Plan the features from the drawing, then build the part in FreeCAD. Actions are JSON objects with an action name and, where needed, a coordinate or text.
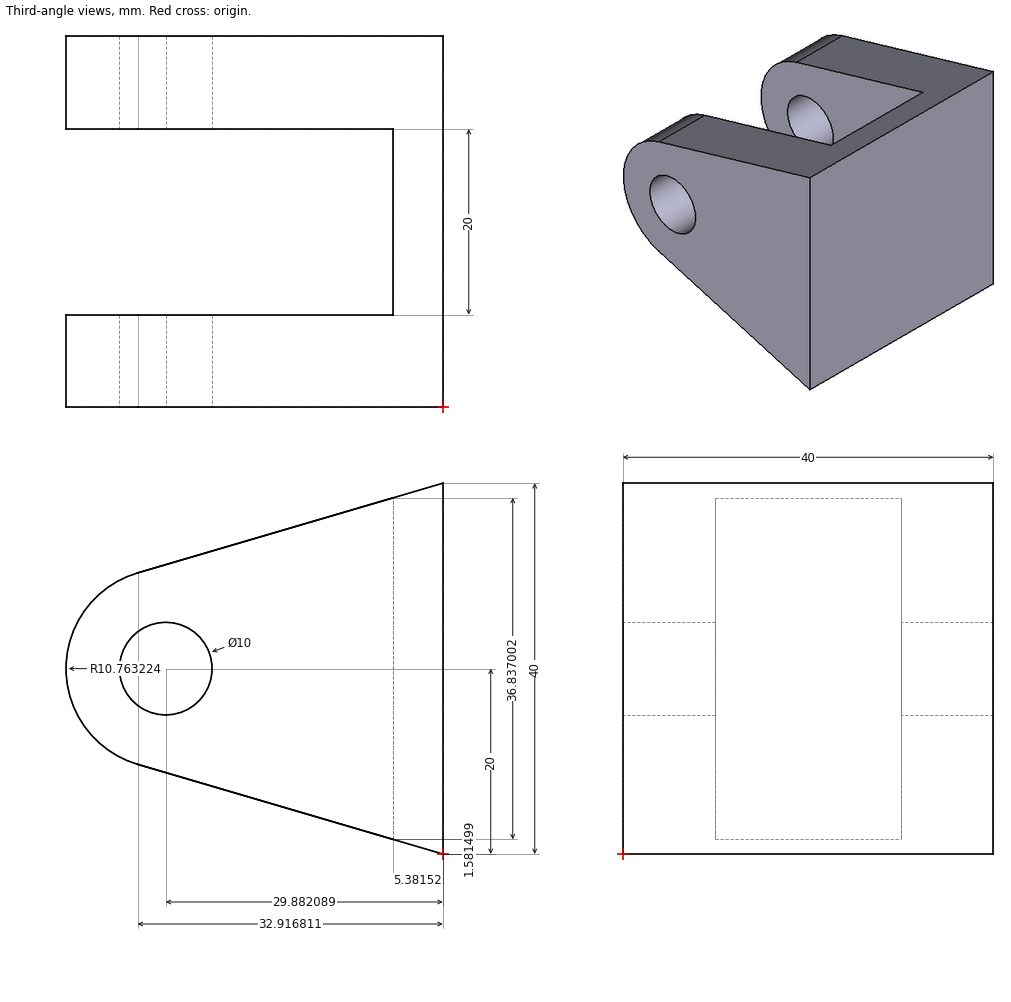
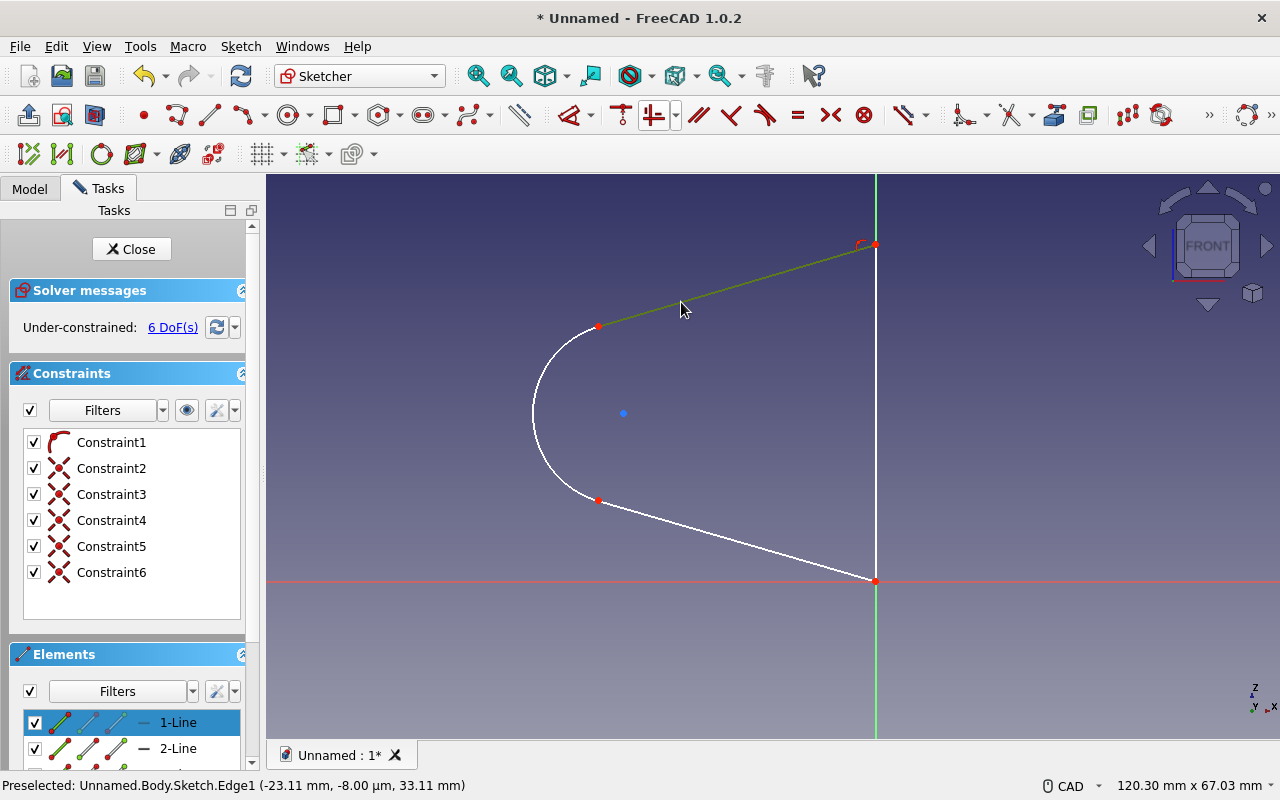
{"action": "left_click", "coordinate": [545, 369]}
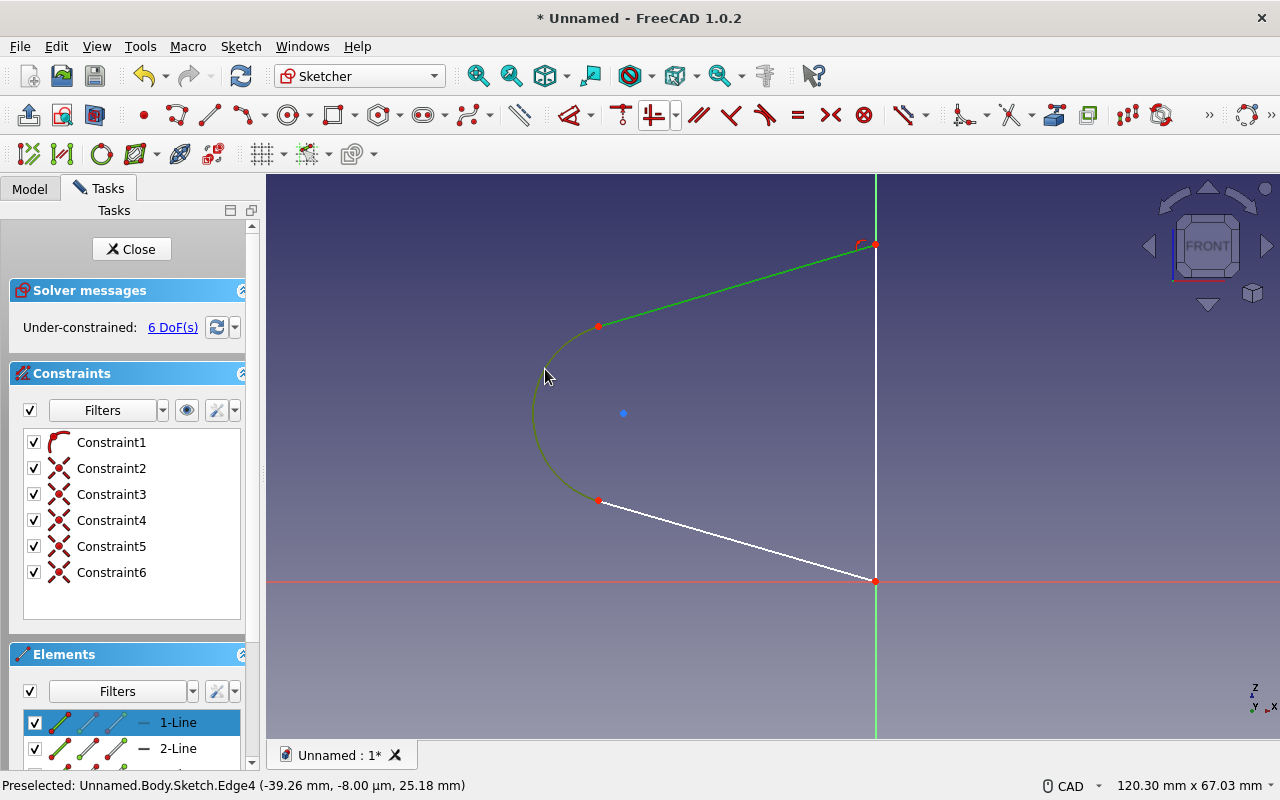
{"action": "left_click", "coordinate": [765, 116]}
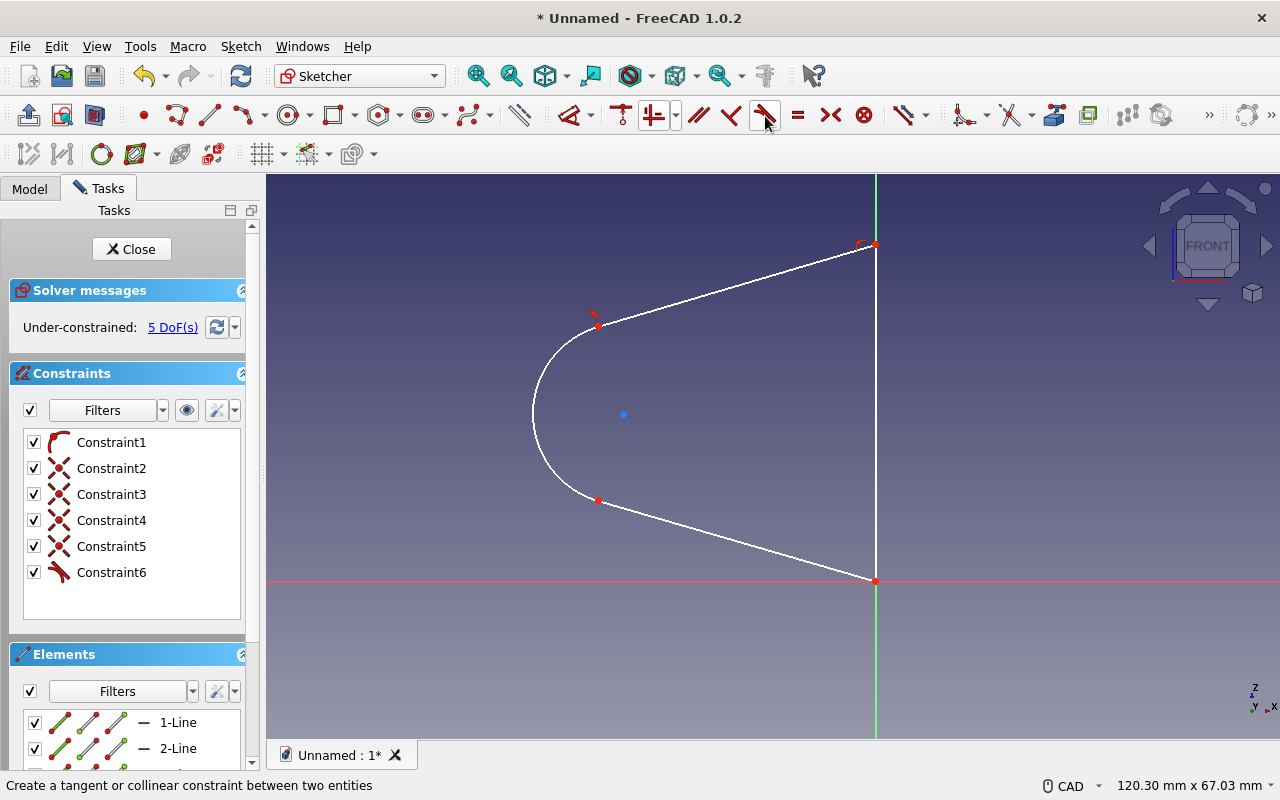
{"action": "left_click", "coordinate": [792, 557]}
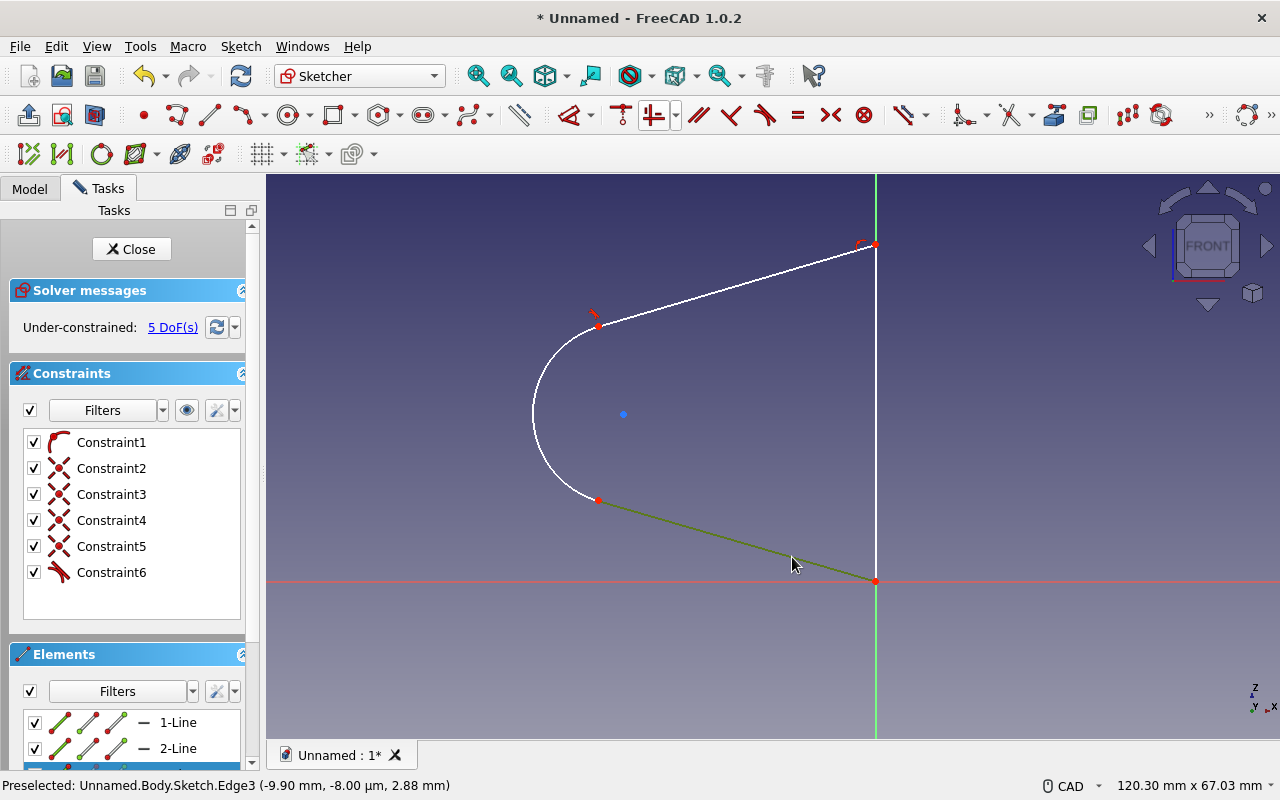
{"action": "left_click", "coordinate": [545, 369]}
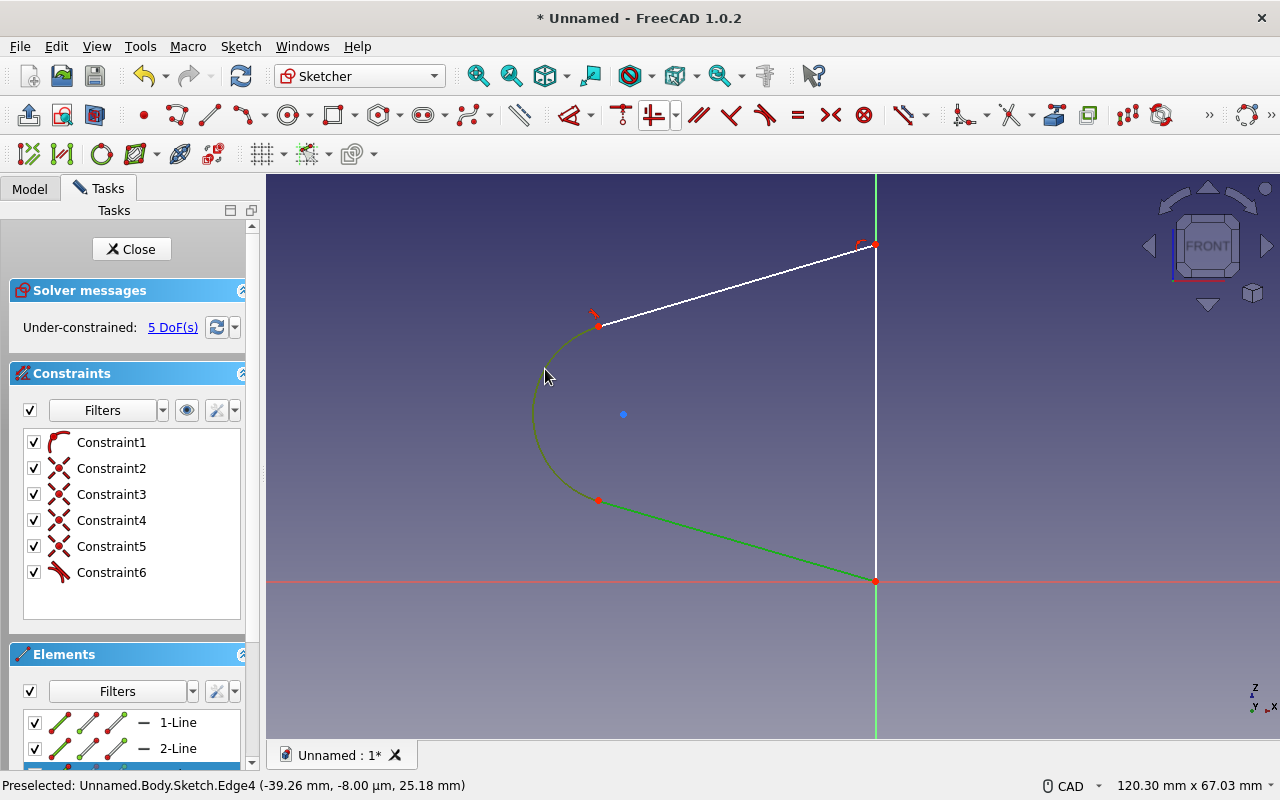
{"action": "left_click", "coordinate": [765, 116]}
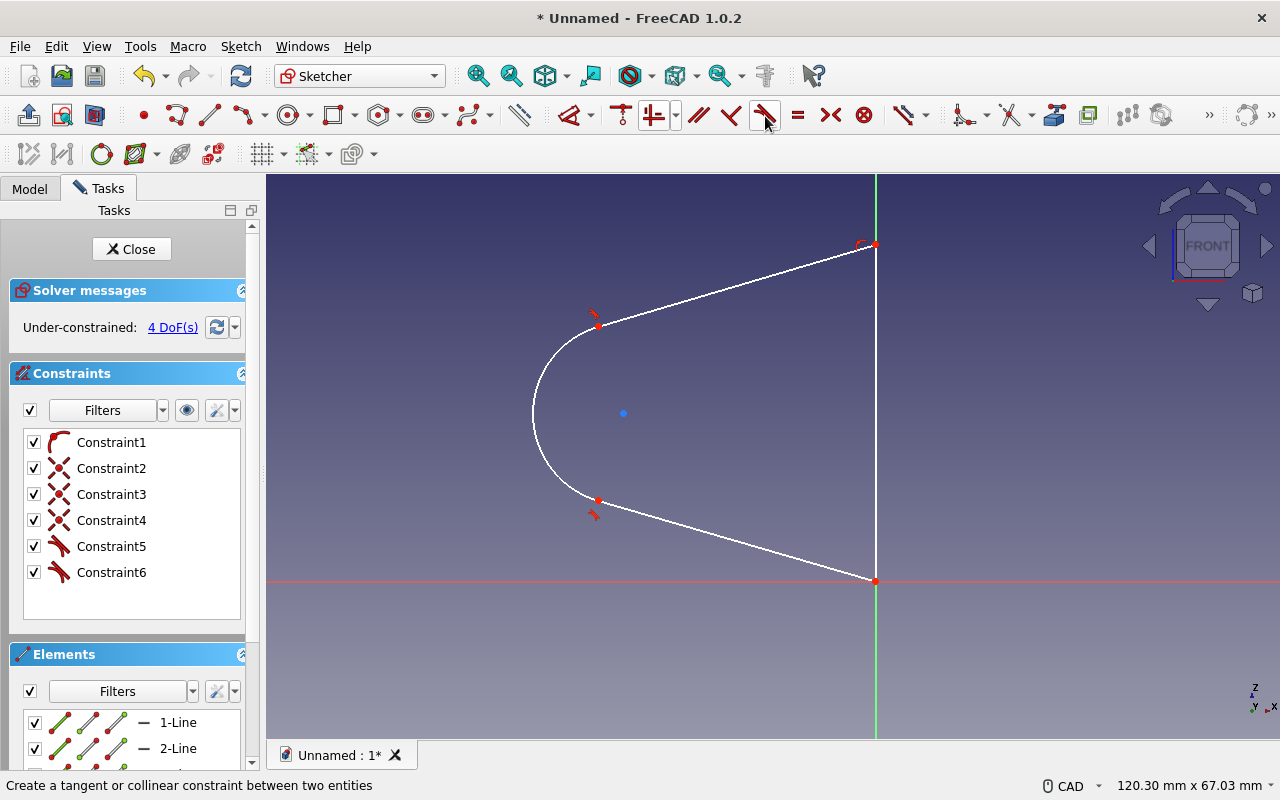
{"action": "left_click", "coordinate": [568, 116]}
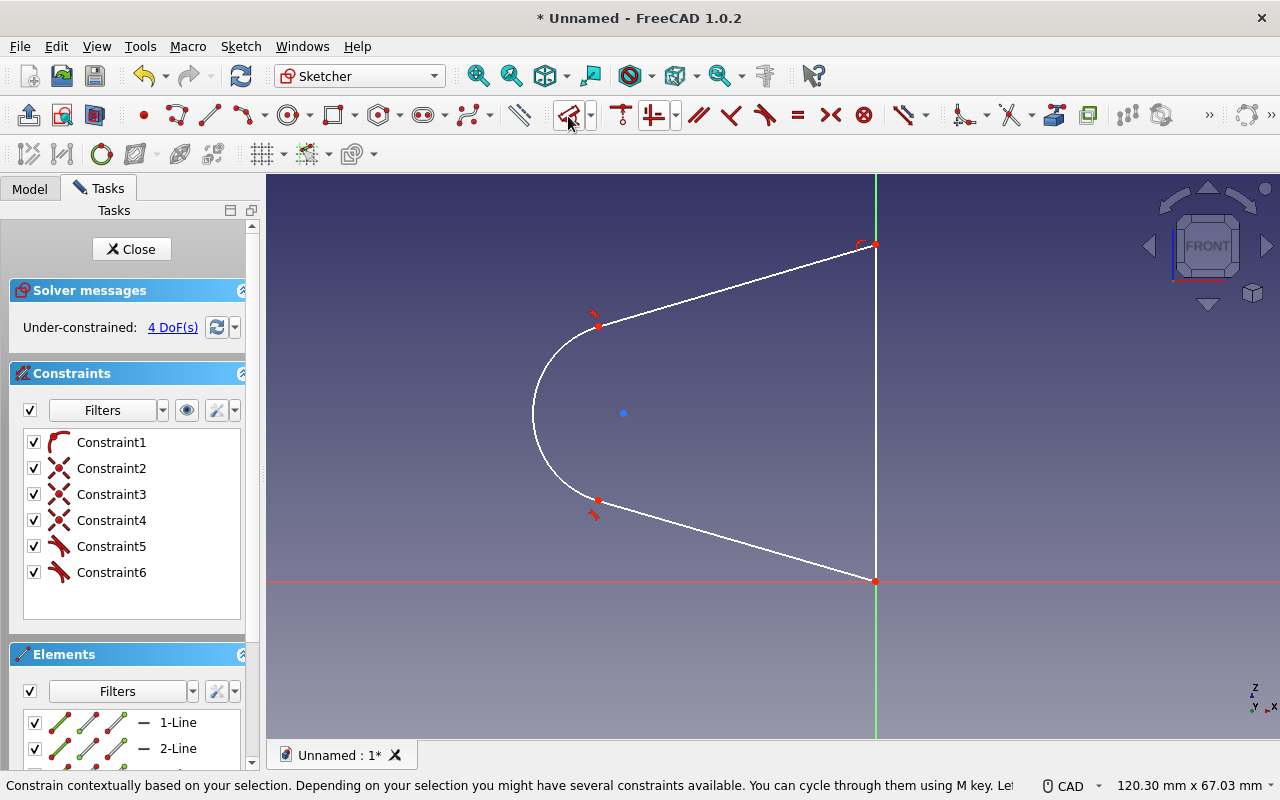
{"action": "left_click", "coordinate": [545, 370]}
{"action": "left_click", "coordinate": [517, 354]}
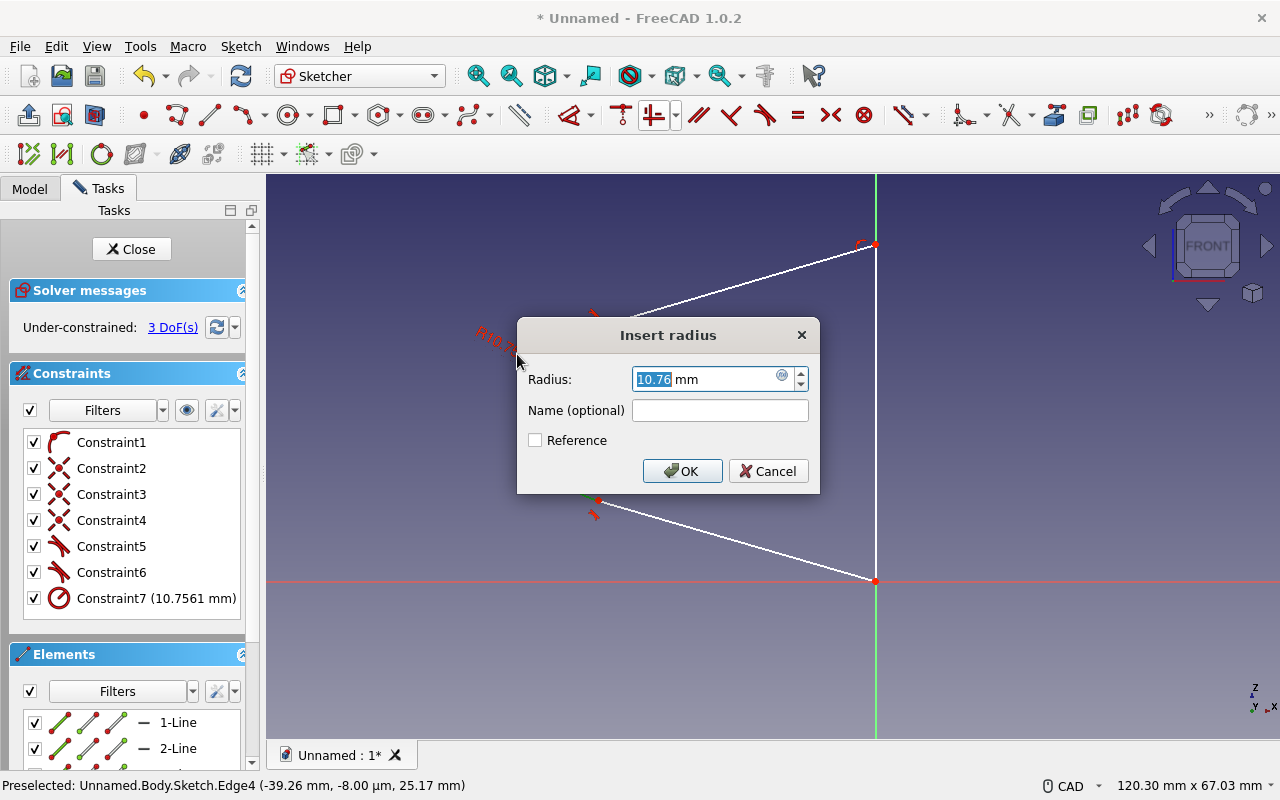
{"action": "type", "text": "10.763224"}
{"action": "key", "text": "Return"}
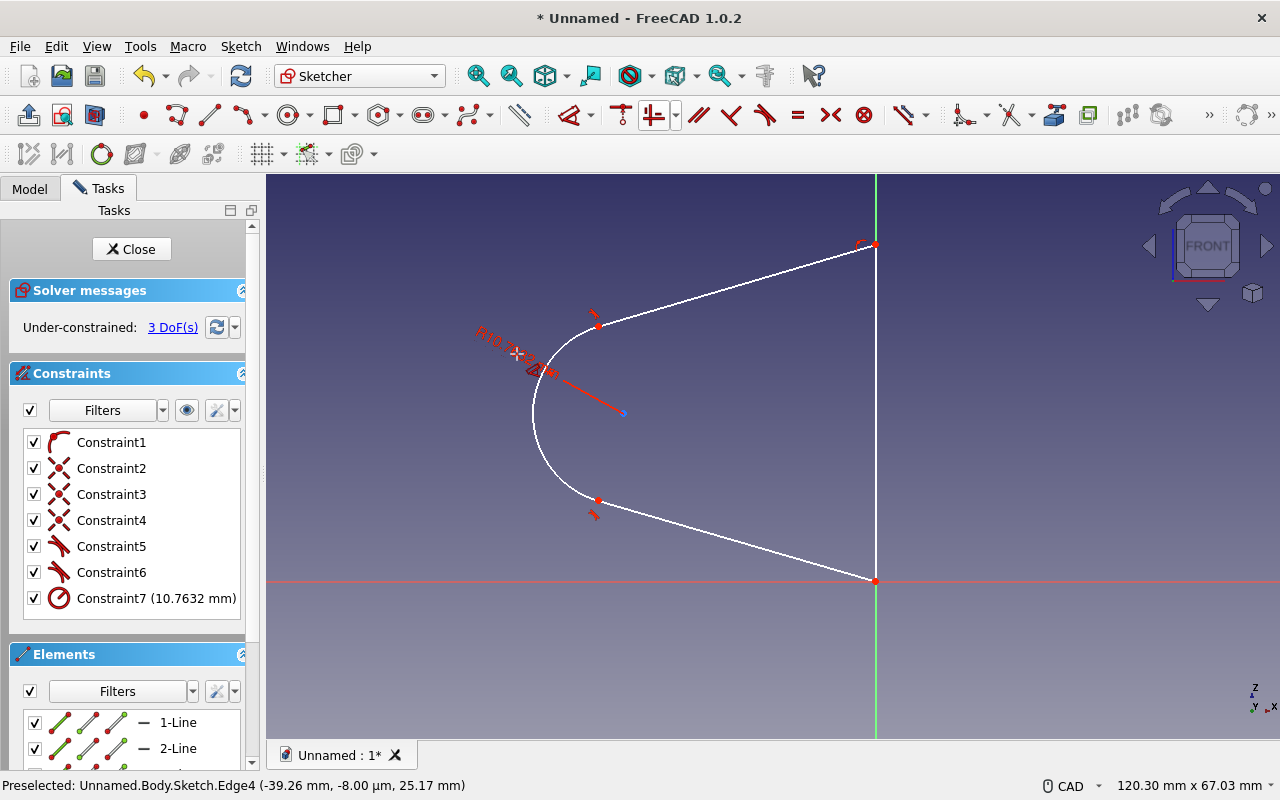
{"action": "left_click", "coordinate": [876, 346]}
{"action": "left_click", "coordinate": [910, 413]}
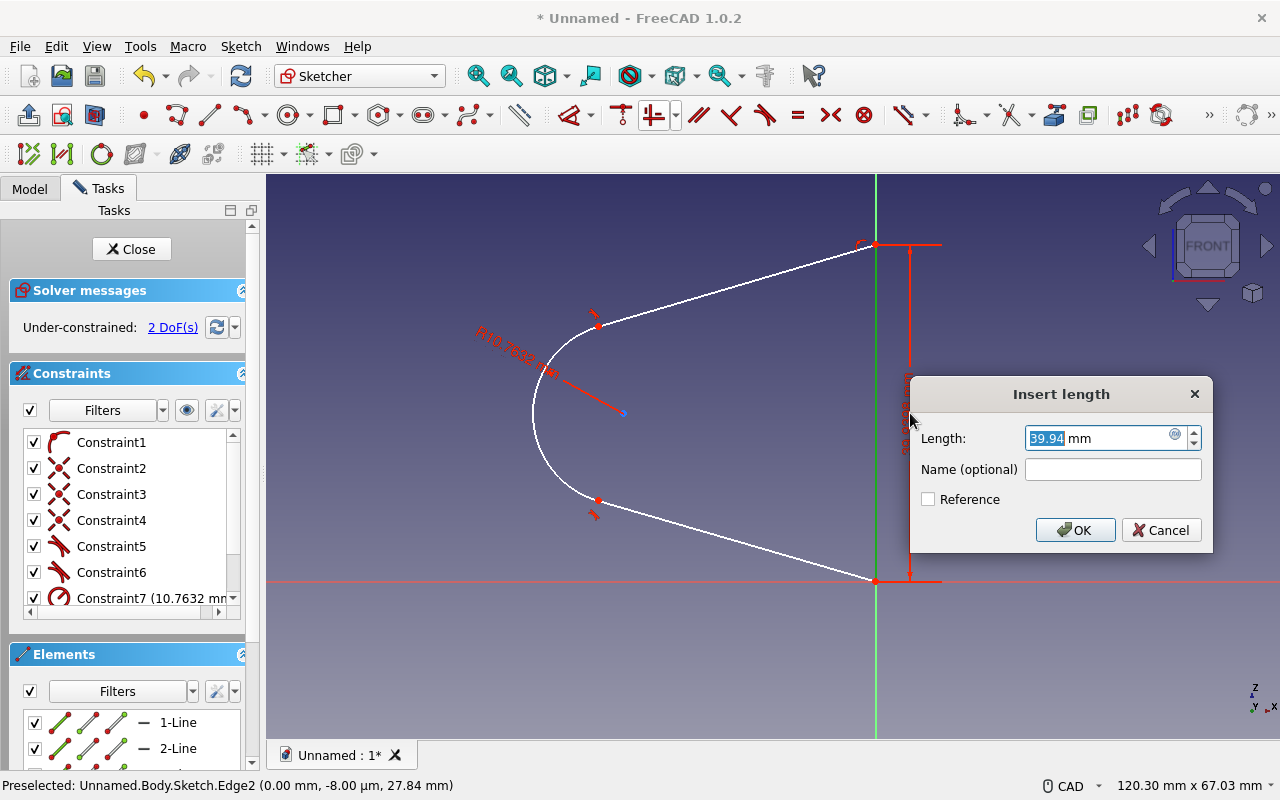
{"action": "type", "text": "40"}
{"action": "key", "text": "Return"}